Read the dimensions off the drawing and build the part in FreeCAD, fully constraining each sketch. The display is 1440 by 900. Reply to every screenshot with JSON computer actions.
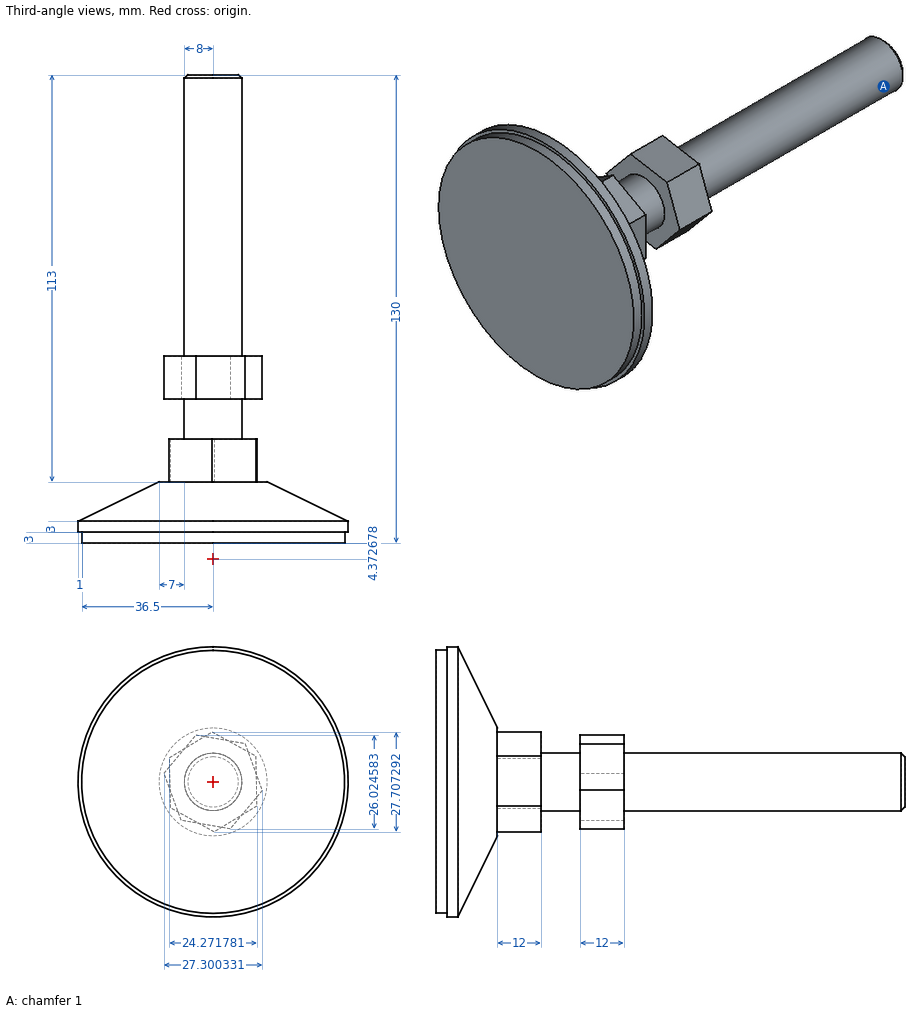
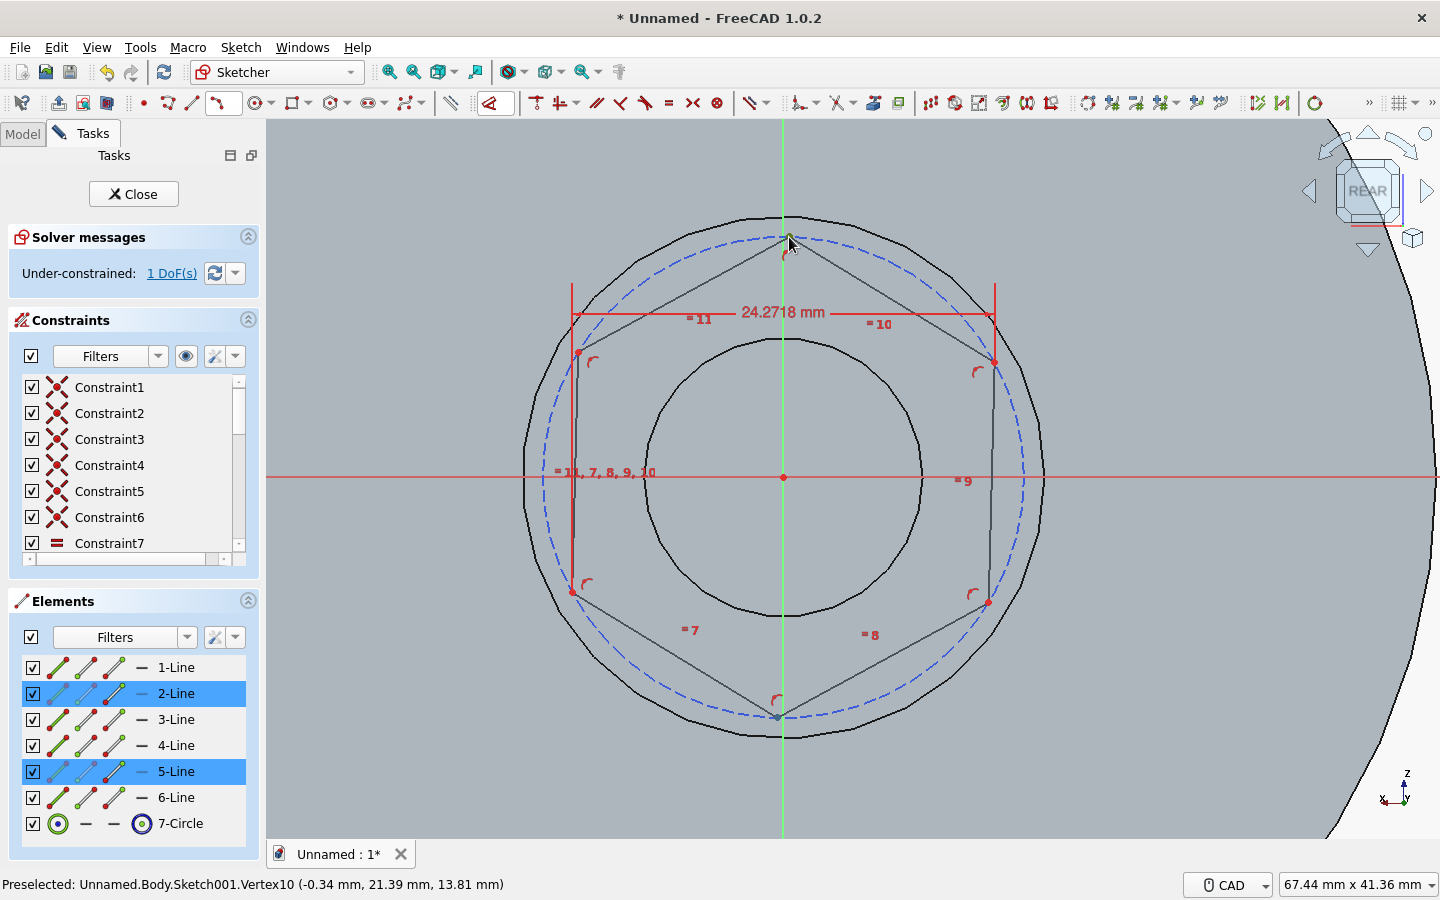
{"action": "left_click", "coordinate": [508, 104]}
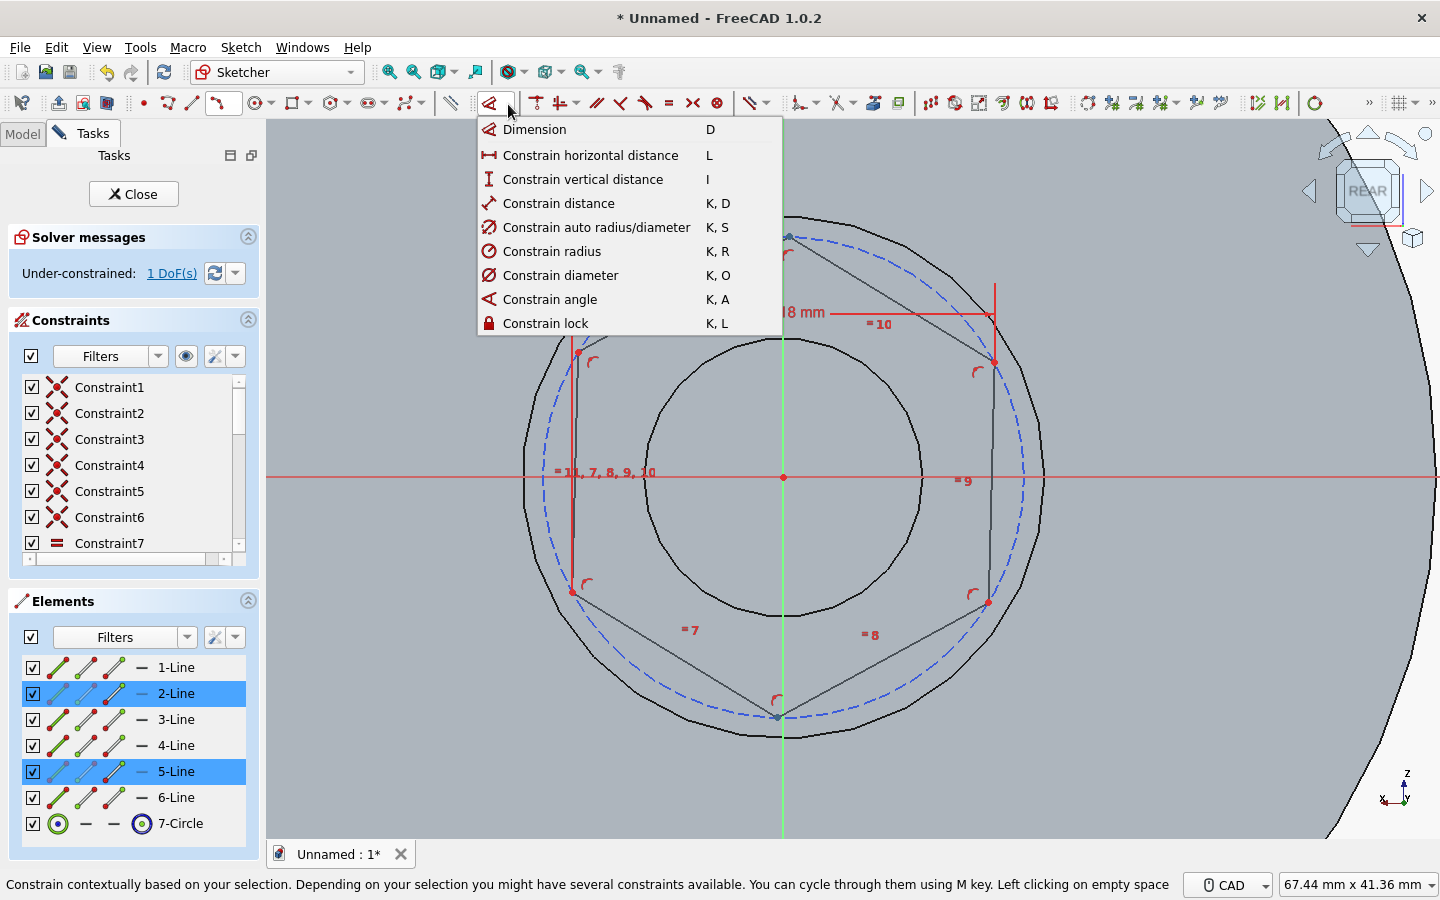
{"action": "left_click", "coordinate": [630, 179]}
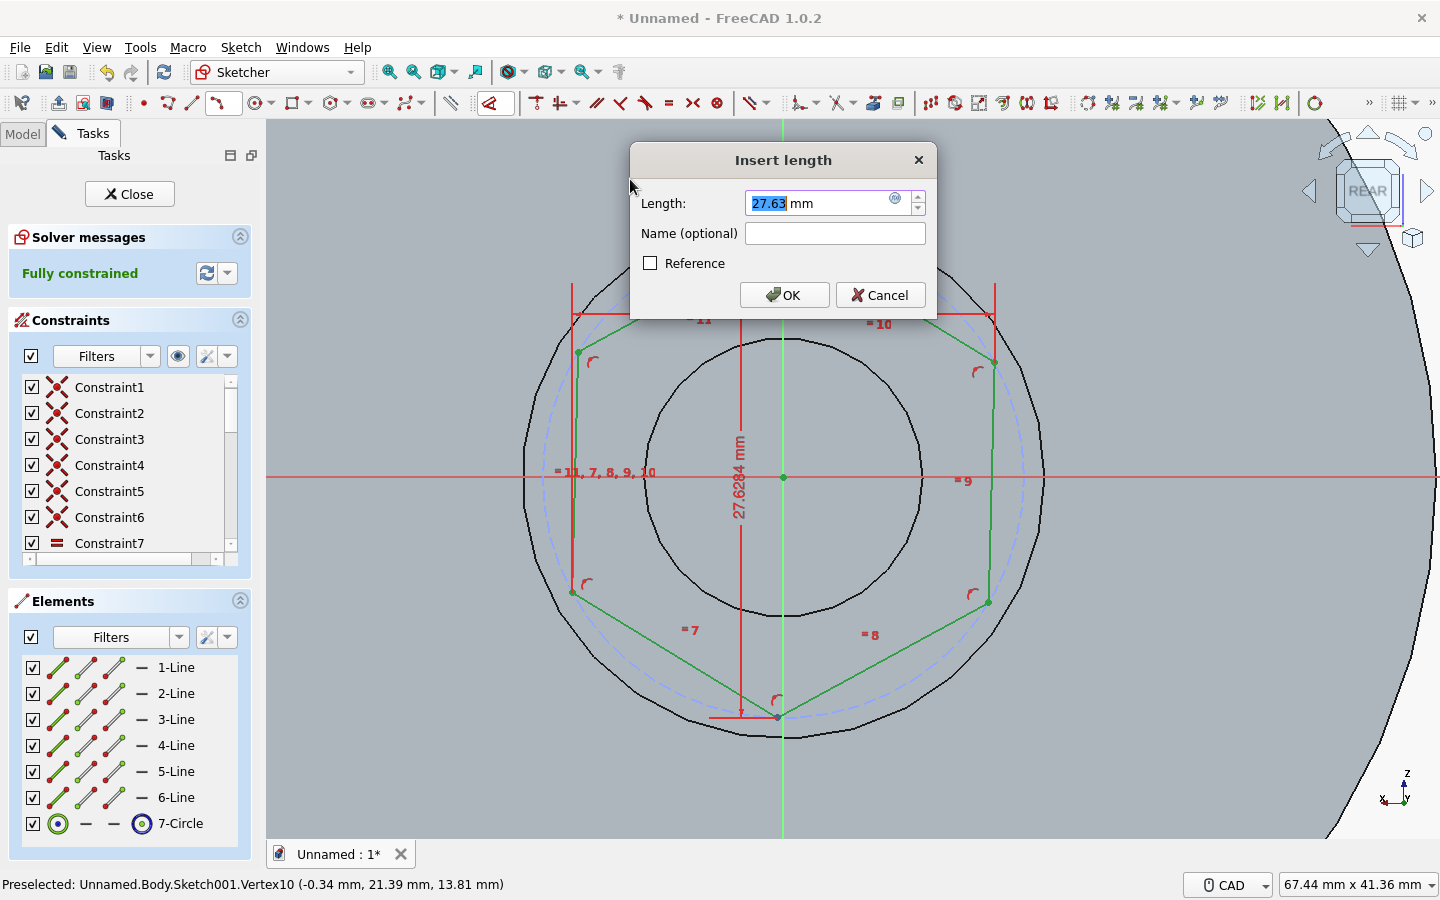
{"action": "type", "text": "27.707292"}
{"action": "key", "text": "Return"}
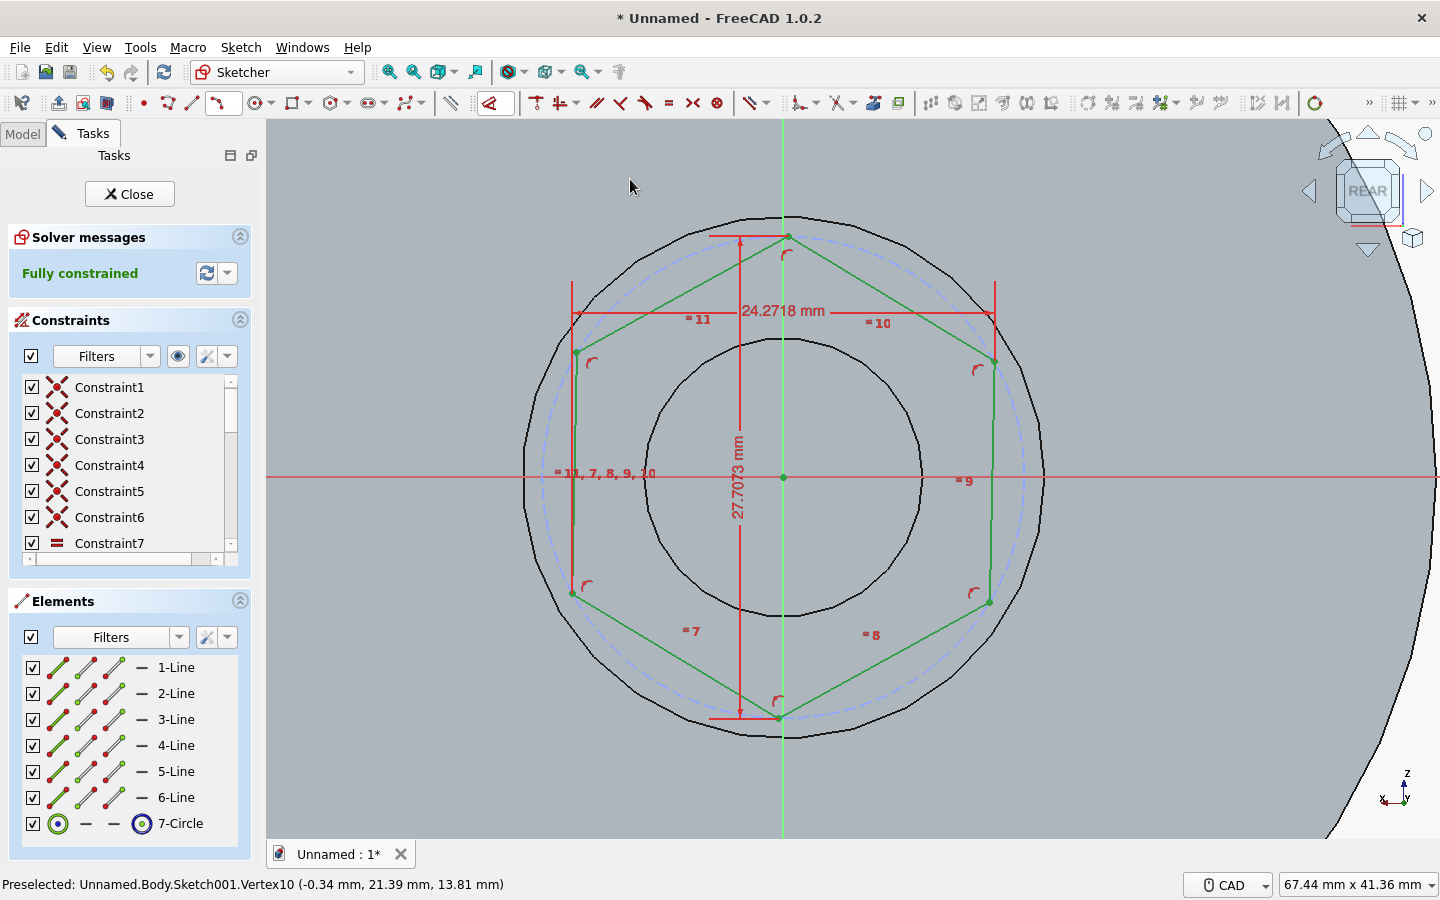
{"action": "left_click", "coordinate": [130, 194]}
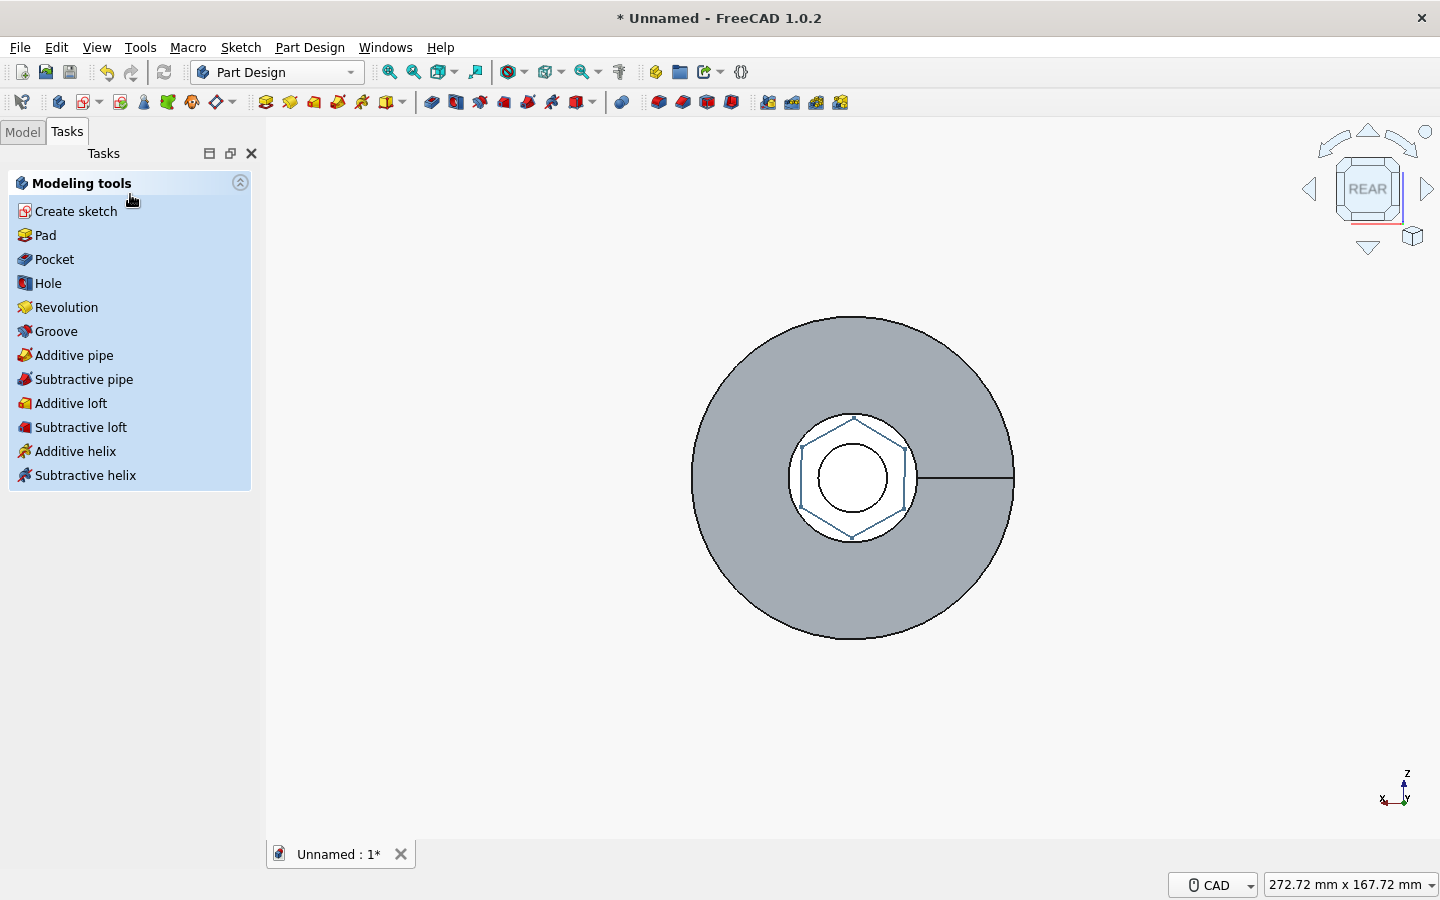
{"action": "left_click", "coordinate": [266, 102]}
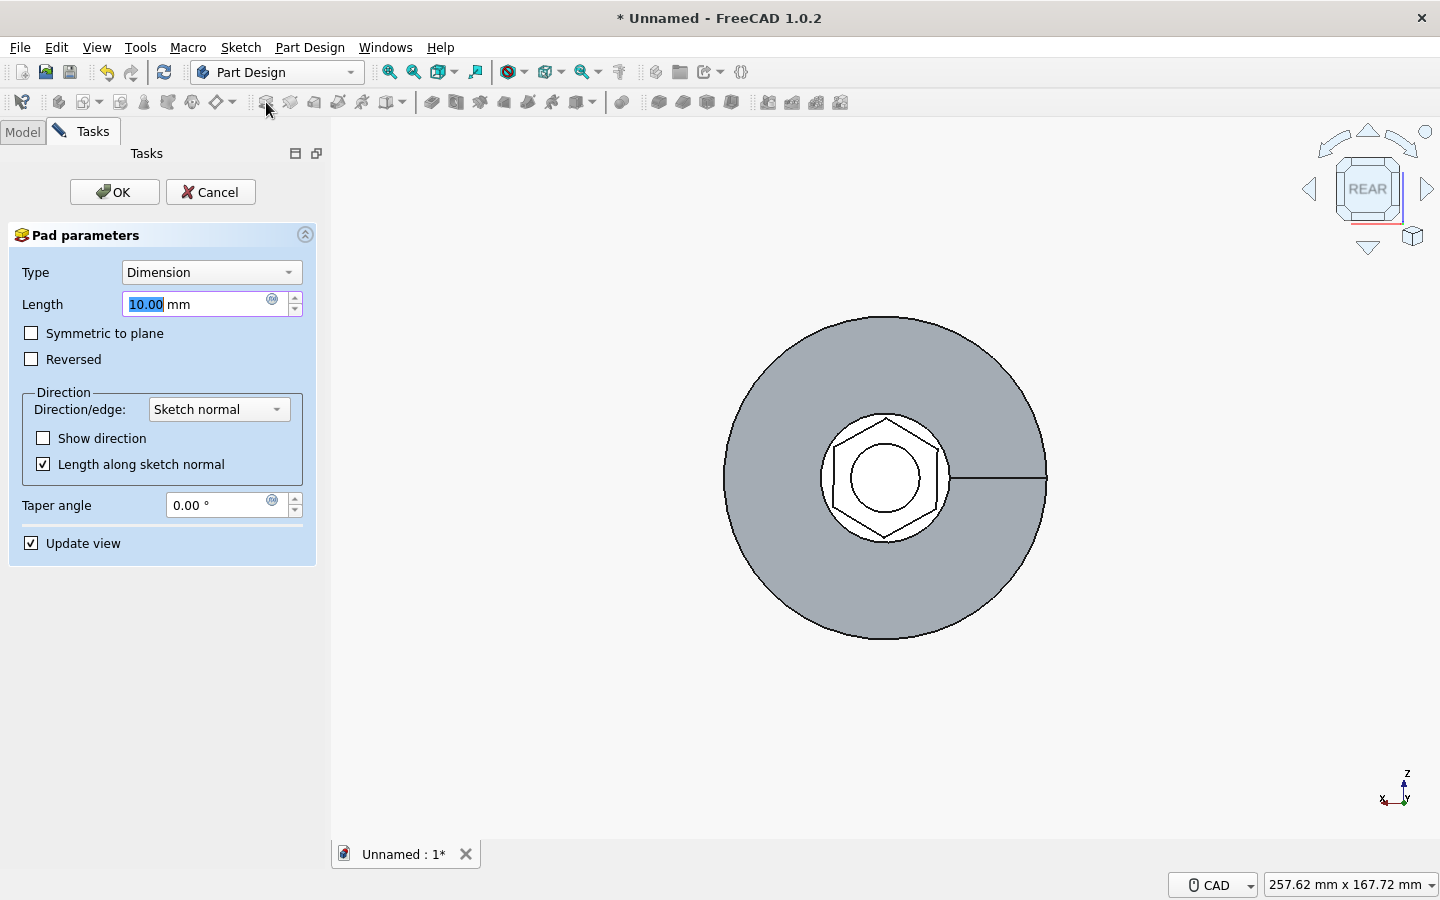
{"action": "type", "text": "12"}
{"action": "key", "text": "Tab"}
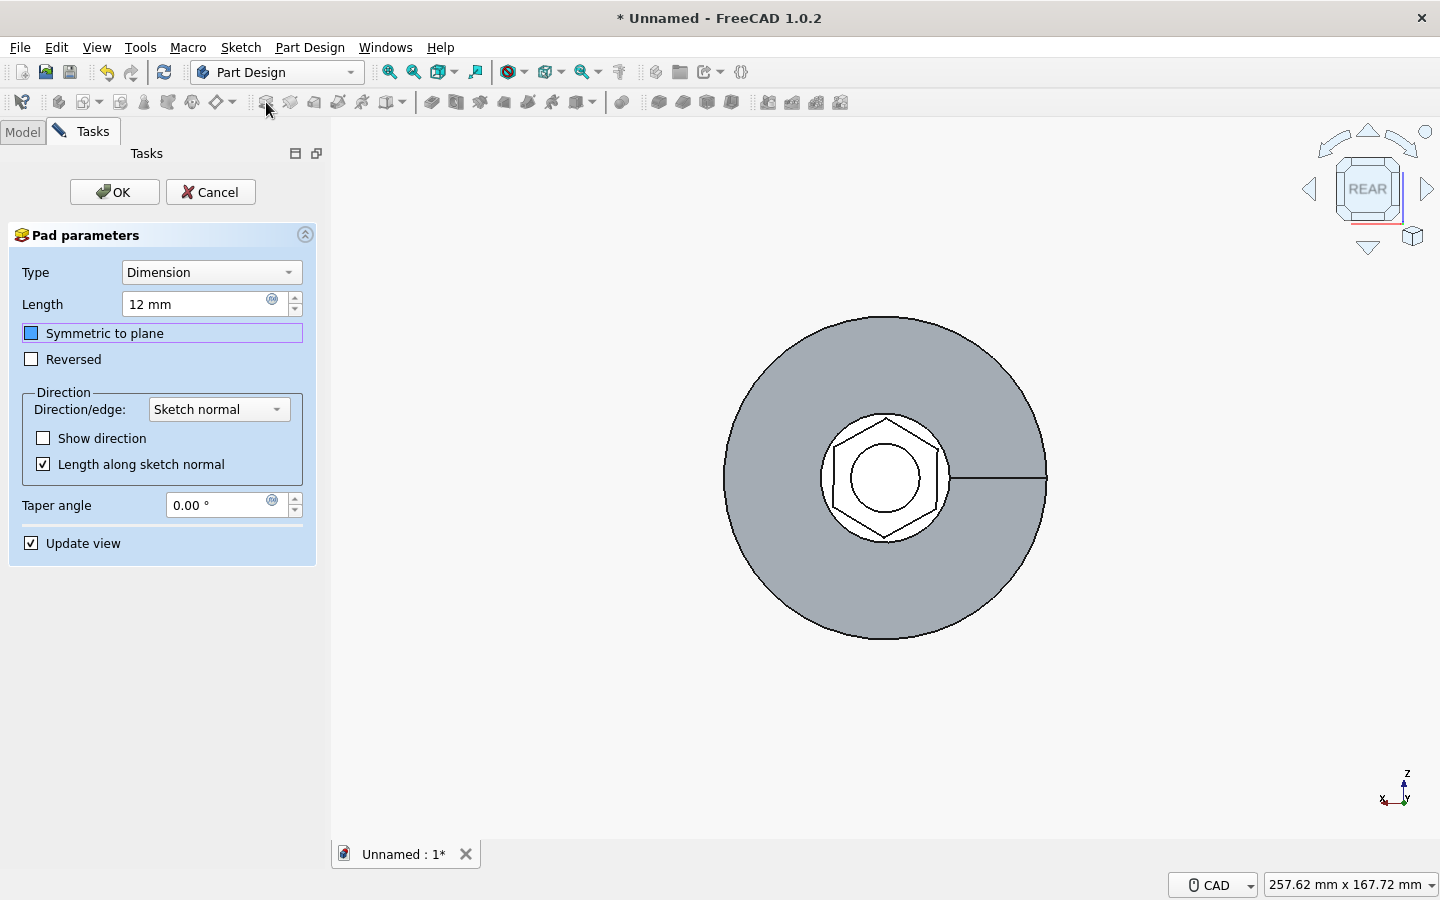
{"action": "left_click", "coordinate": [115, 192]}